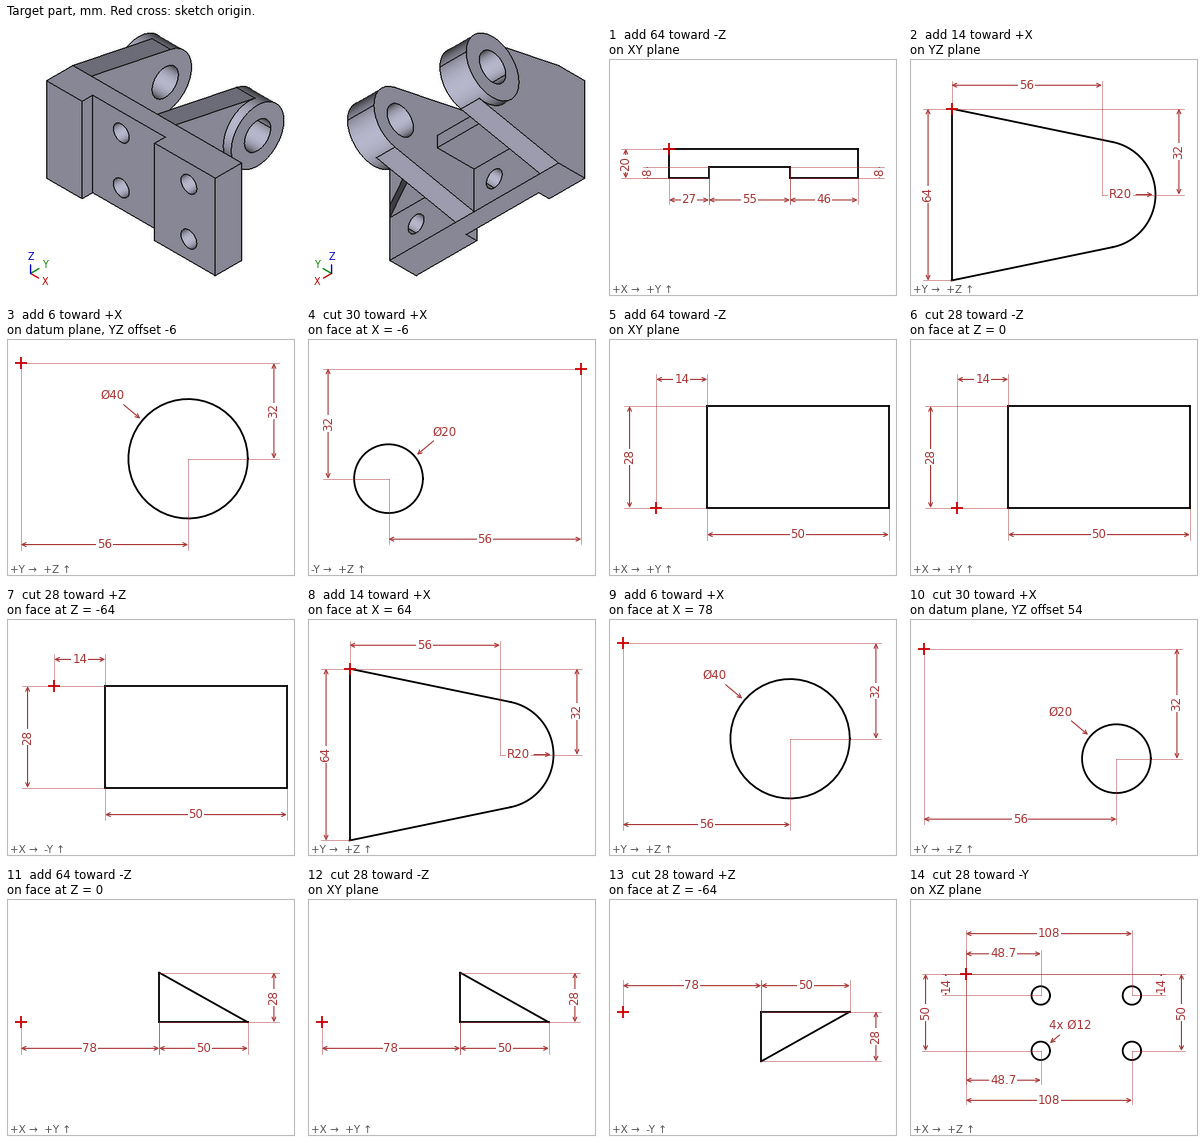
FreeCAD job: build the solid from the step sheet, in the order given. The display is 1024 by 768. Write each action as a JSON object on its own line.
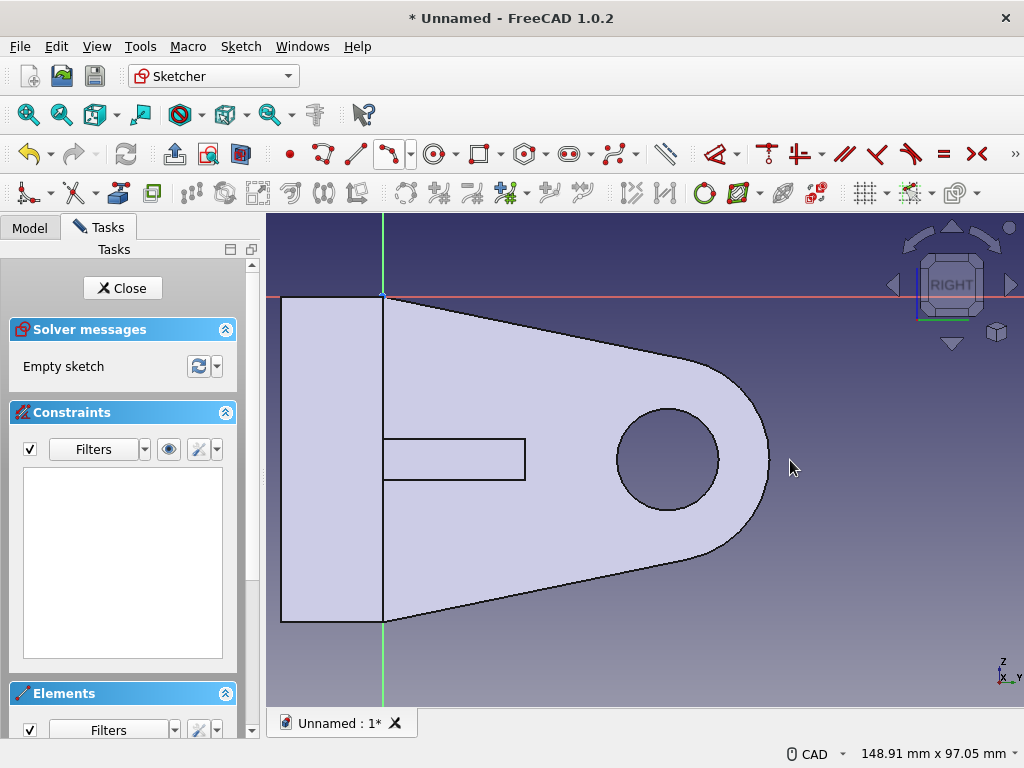
{"action": "left_click", "coordinate": [323, 154]}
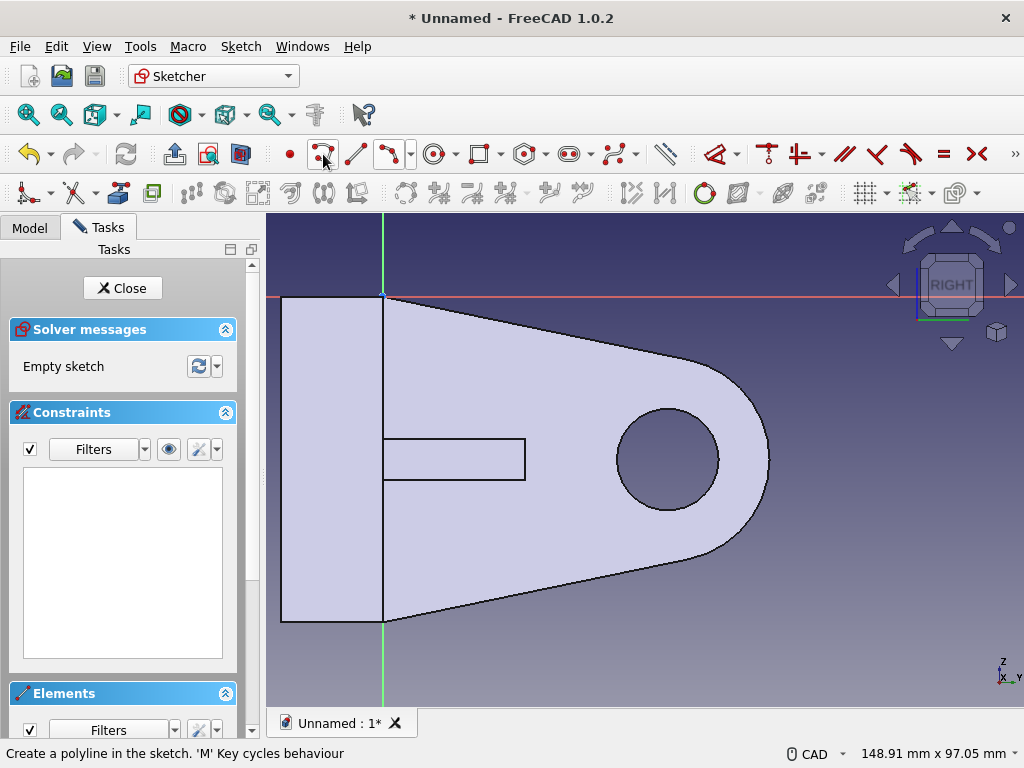
{"action": "left_click", "coordinate": [688, 360]}
{"action": "left_click", "coordinate": [383, 297]}
{"action": "left_click", "coordinate": [392, 622]}
{"action": "left_click", "coordinate": [688, 559]}
{"action": "right_click", "coordinate": [688, 559]}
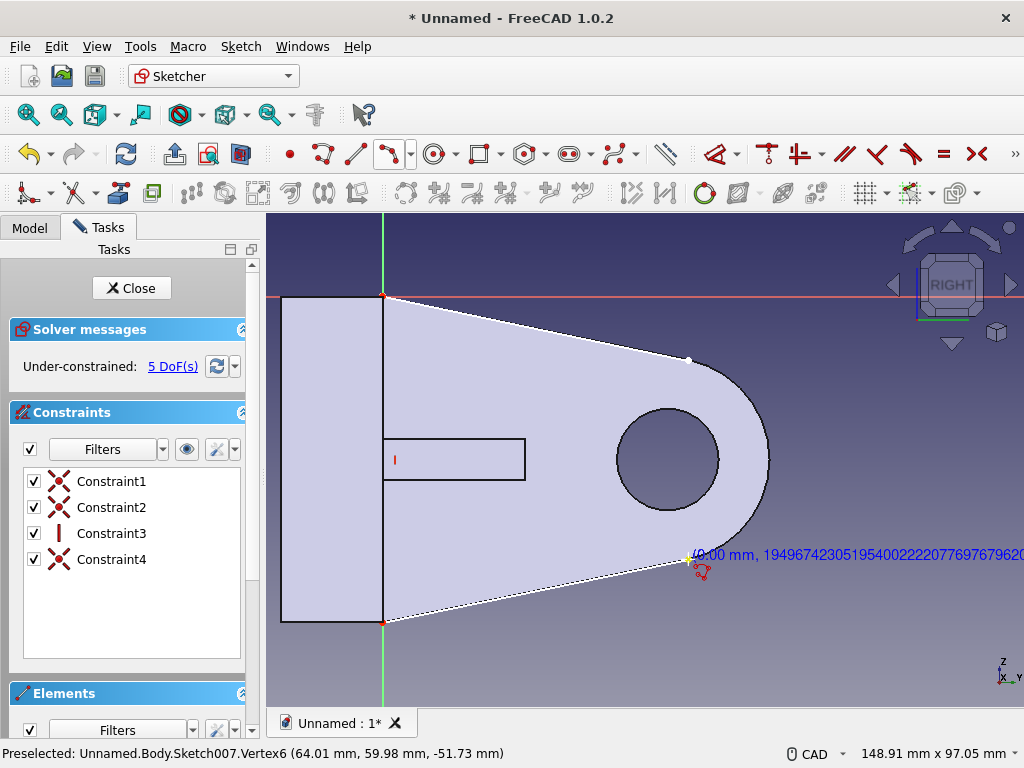
{"action": "left_click", "coordinate": [388, 154]}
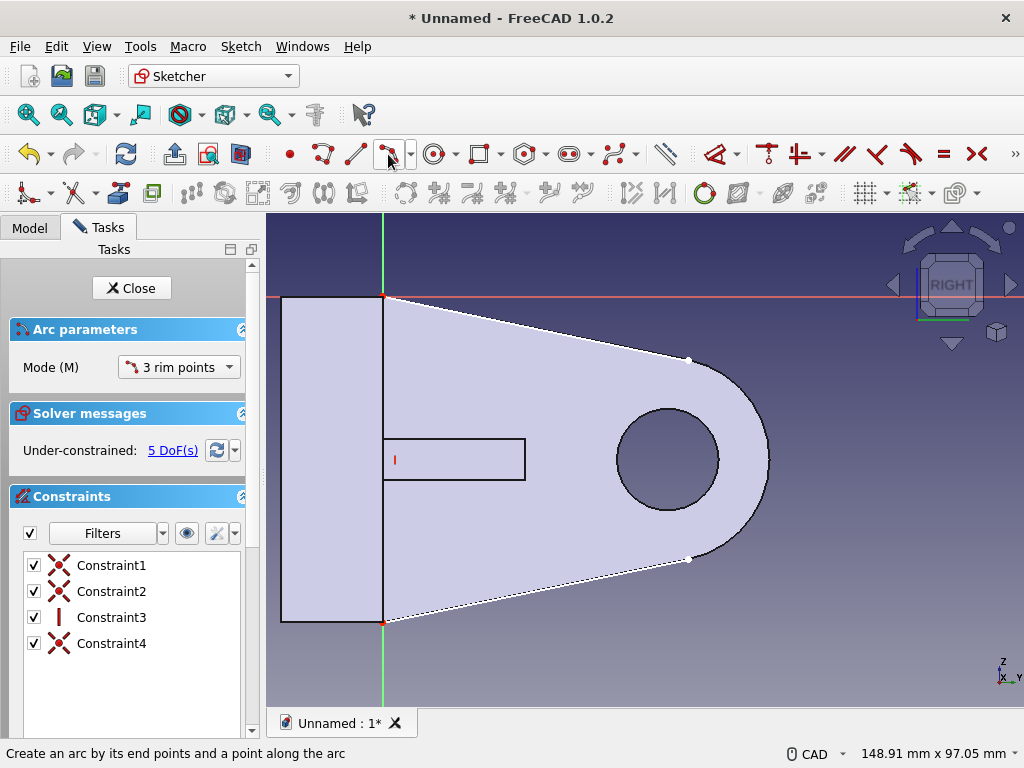
{"action": "left_click", "coordinate": [688, 560]}
{"action": "left_click", "coordinate": [688, 361]}
{"action": "left_click", "coordinate": [770, 460]}
{"action": "key", "text": "Escape"}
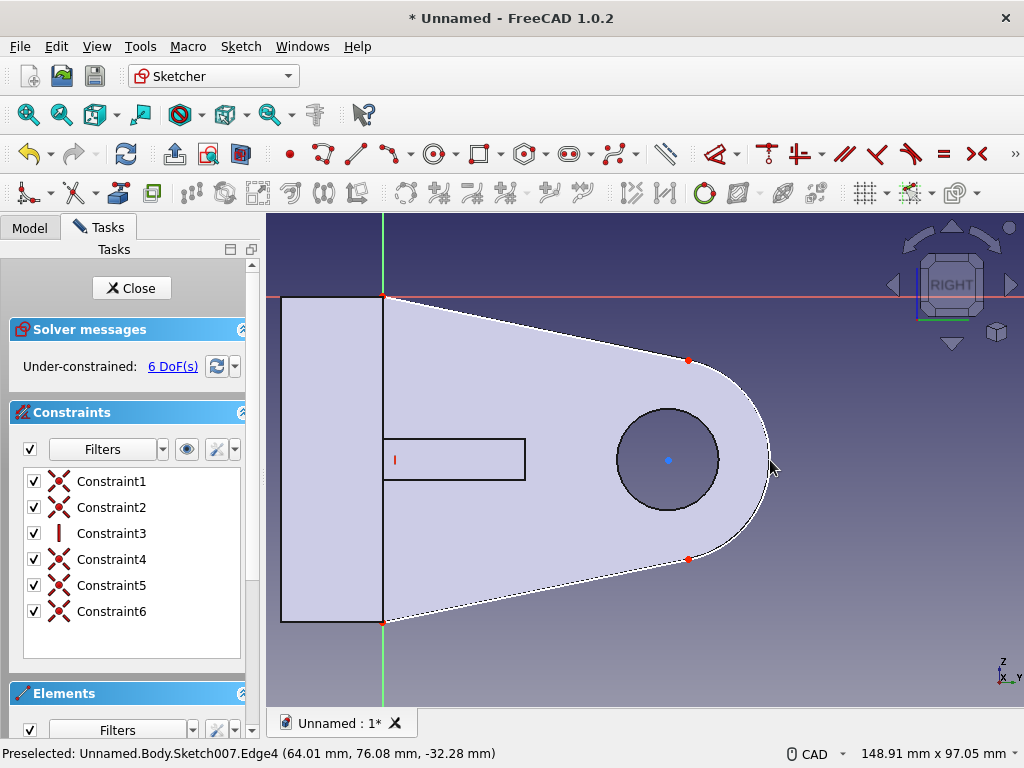
{"action": "left_click", "coordinate": [596, 342]}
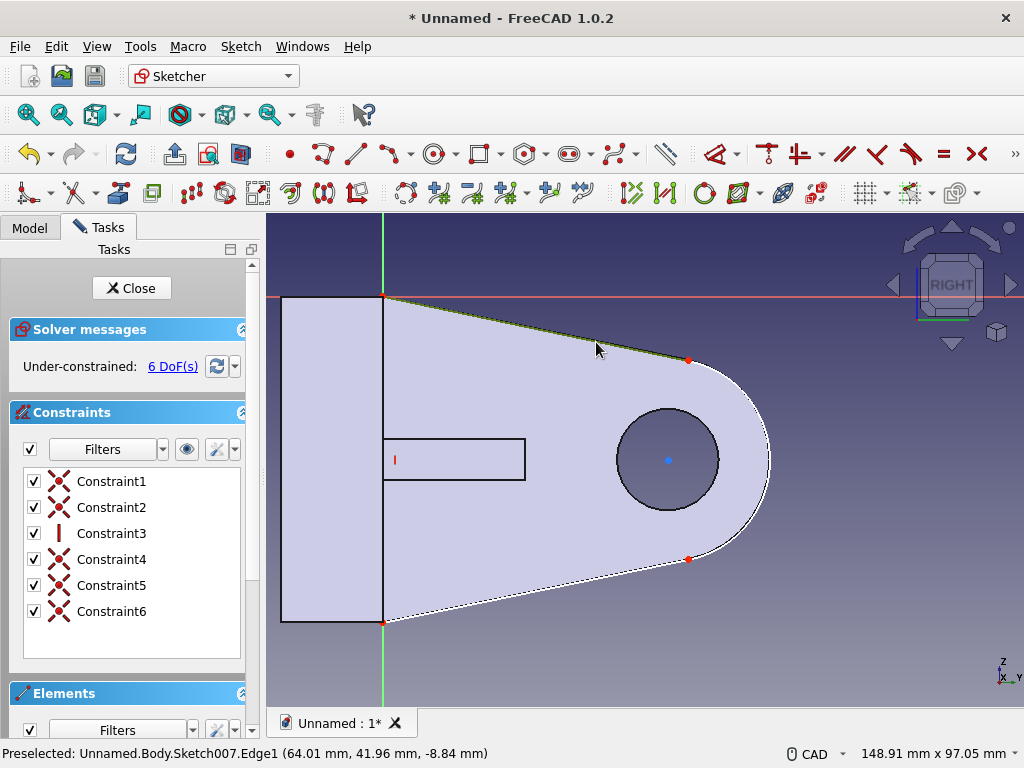
{"action": "left_click", "coordinate": [755, 514]}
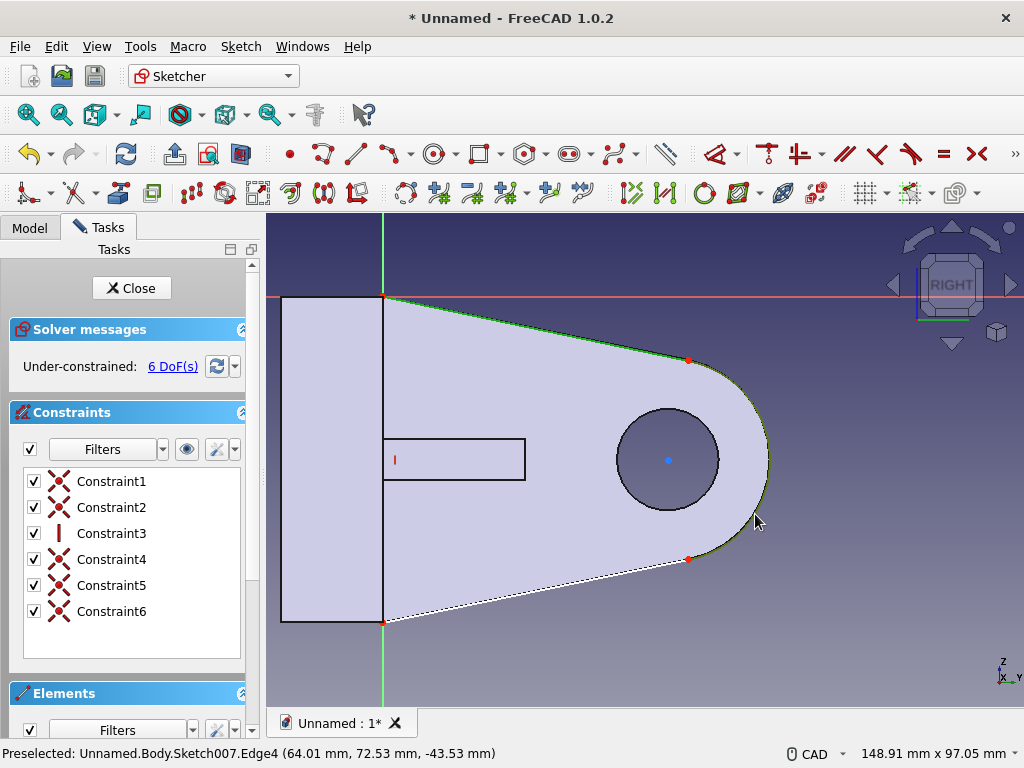
{"action": "left_click", "coordinate": [911, 154]}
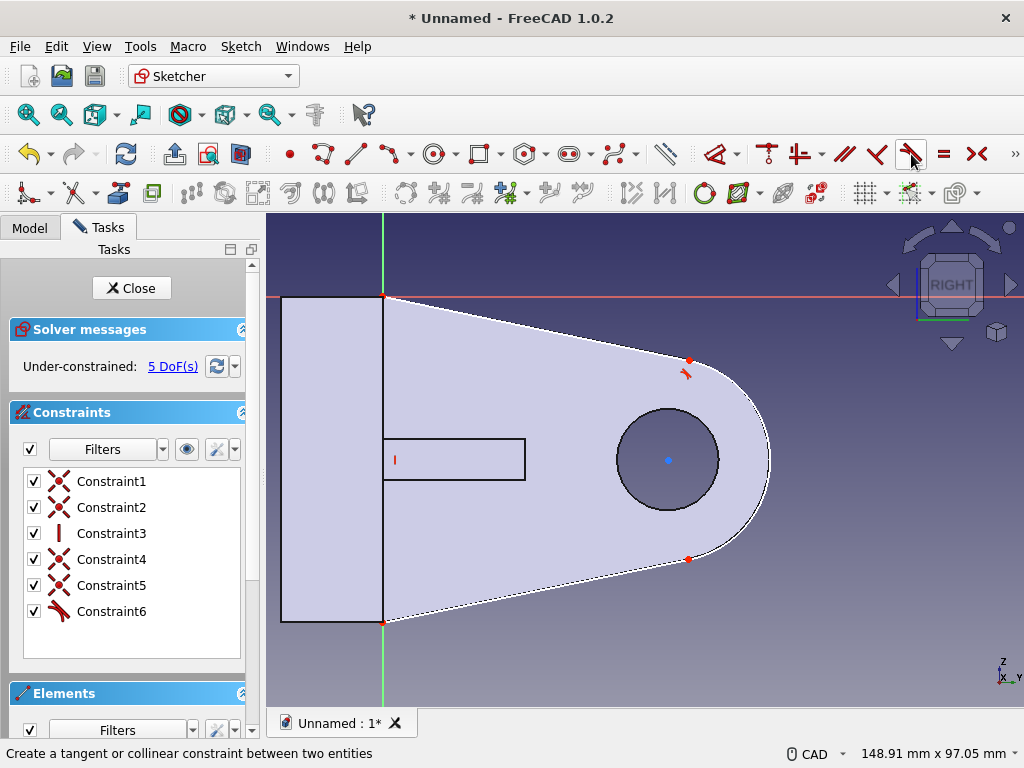
{"action": "left_click", "coordinate": [474, 604]}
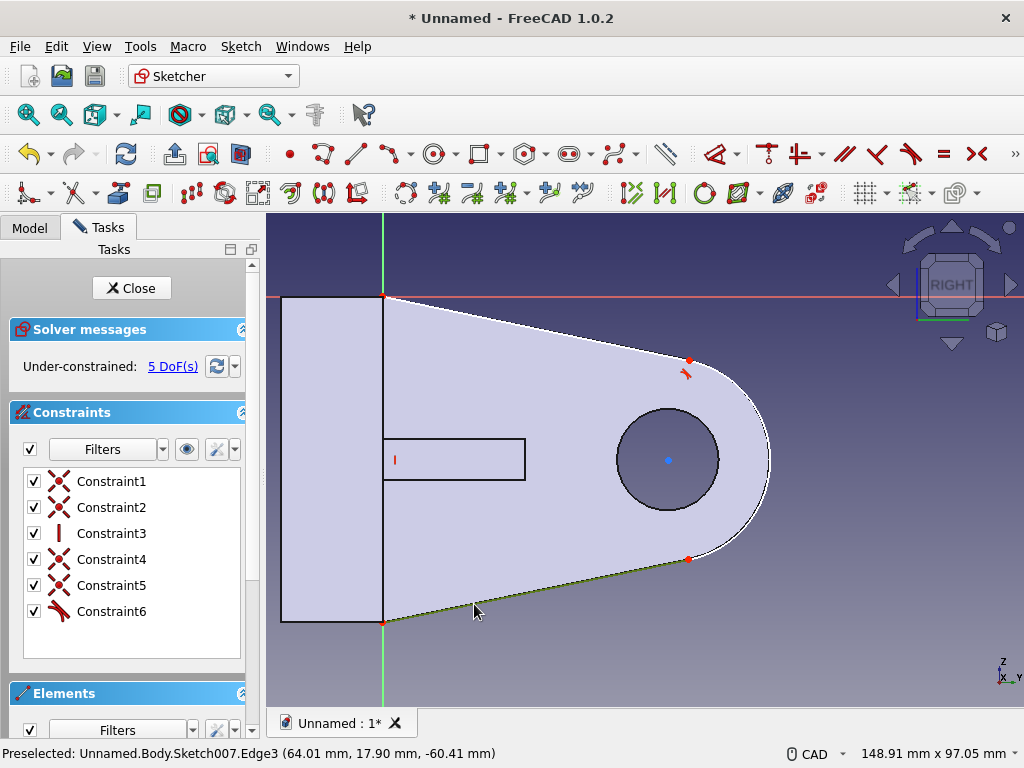
{"action": "left_click", "coordinate": [755, 514]}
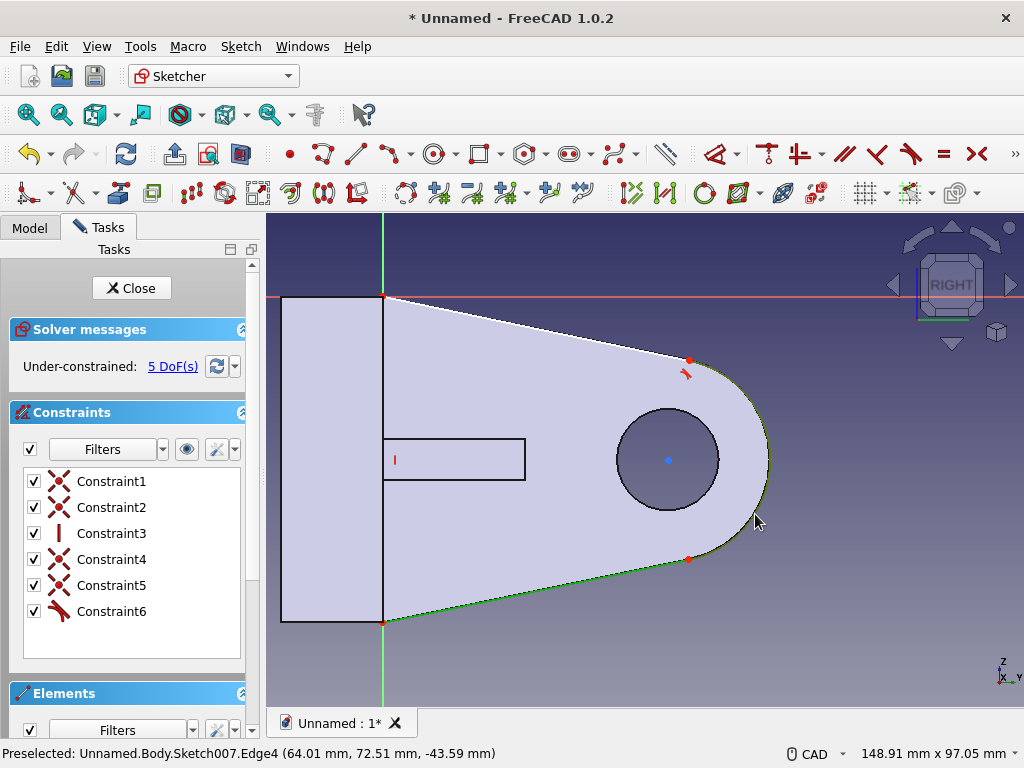
{"action": "left_click", "coordinate": [911, 154]}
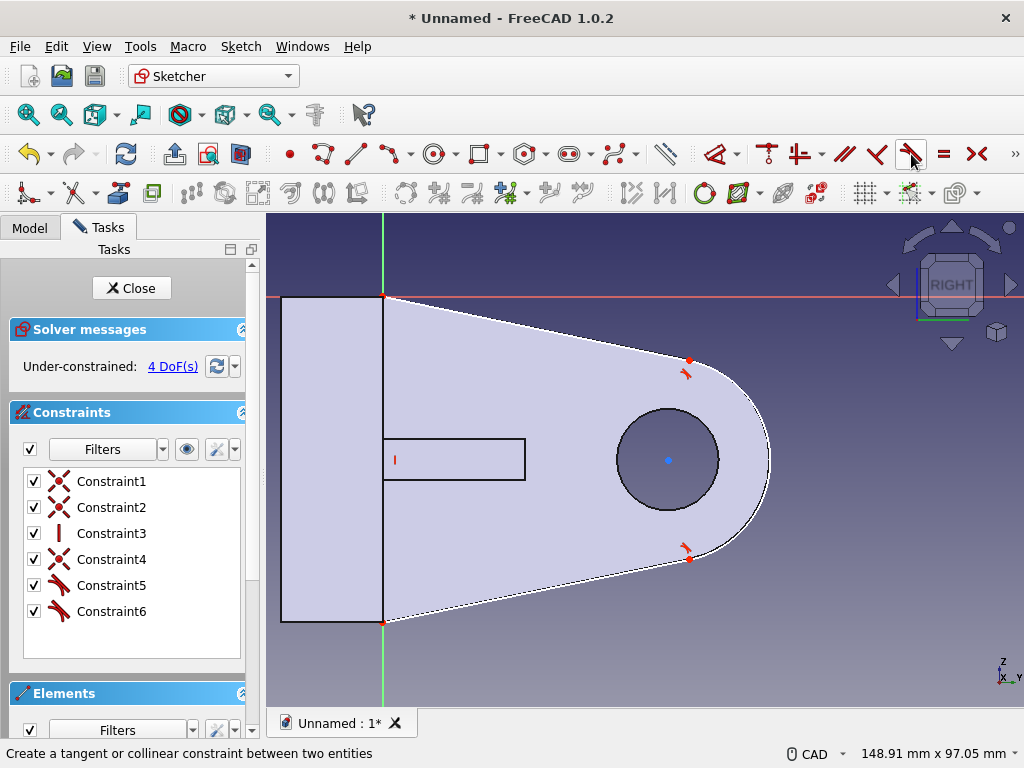
{"action": "left_click", "coordinate": [714, 154]}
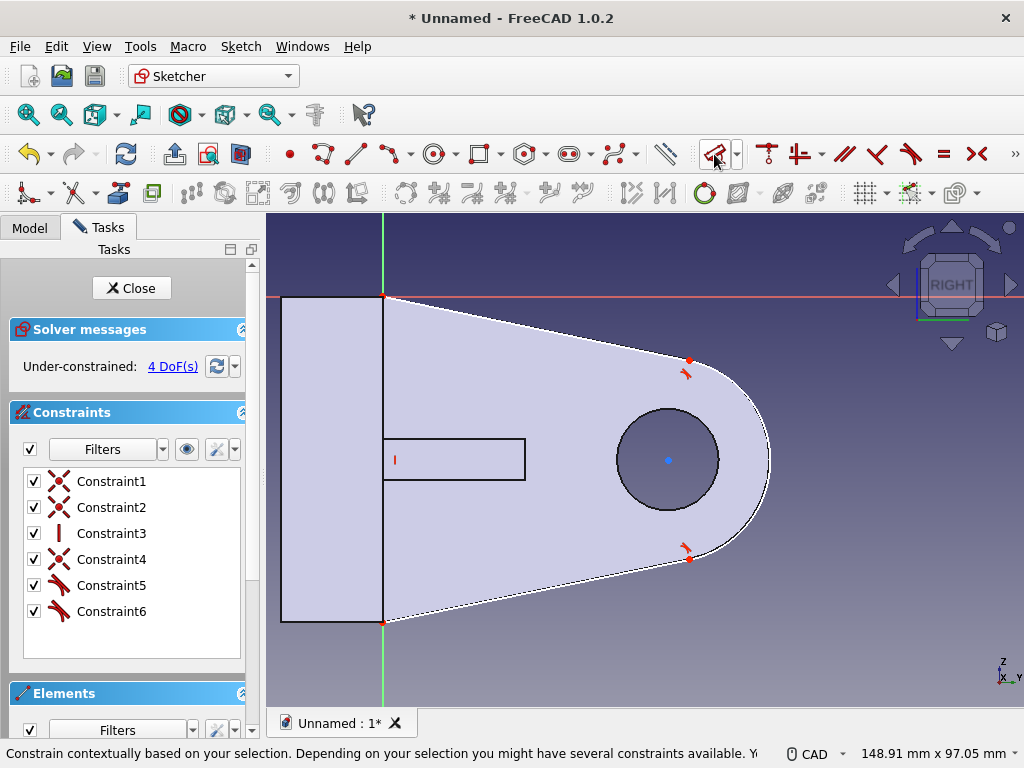
{"action": "left_click", "coordinate": [755, 513]}
{"action": "left_click", "coordinate": [782, 530]}